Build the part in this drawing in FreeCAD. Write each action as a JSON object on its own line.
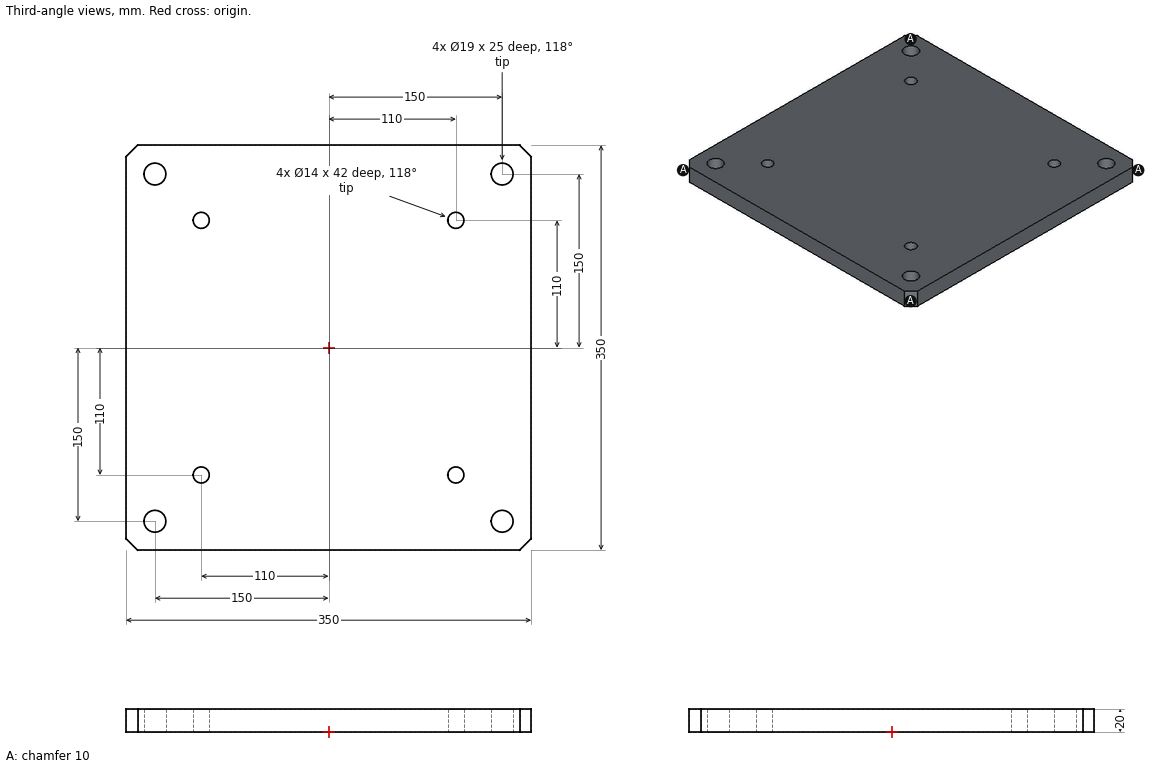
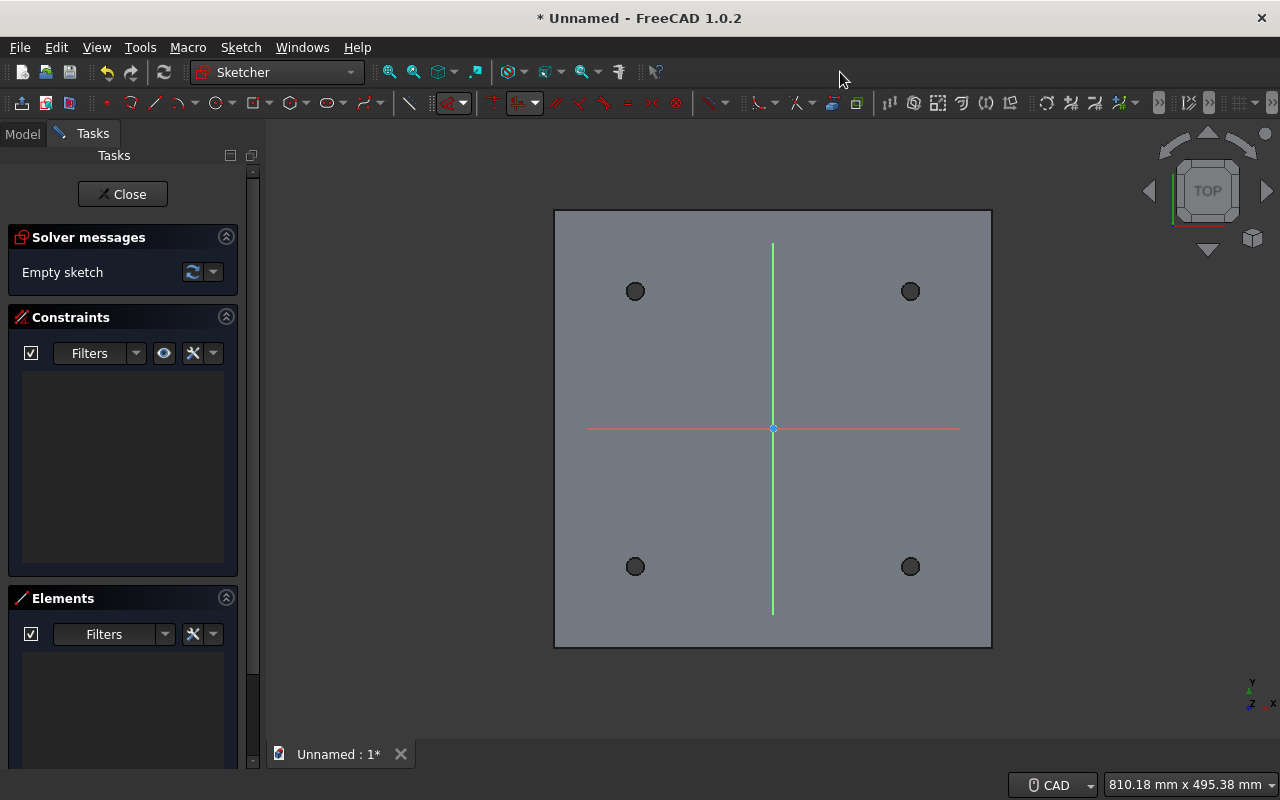
{"action": "left_click", "coordinate": [216, 104]}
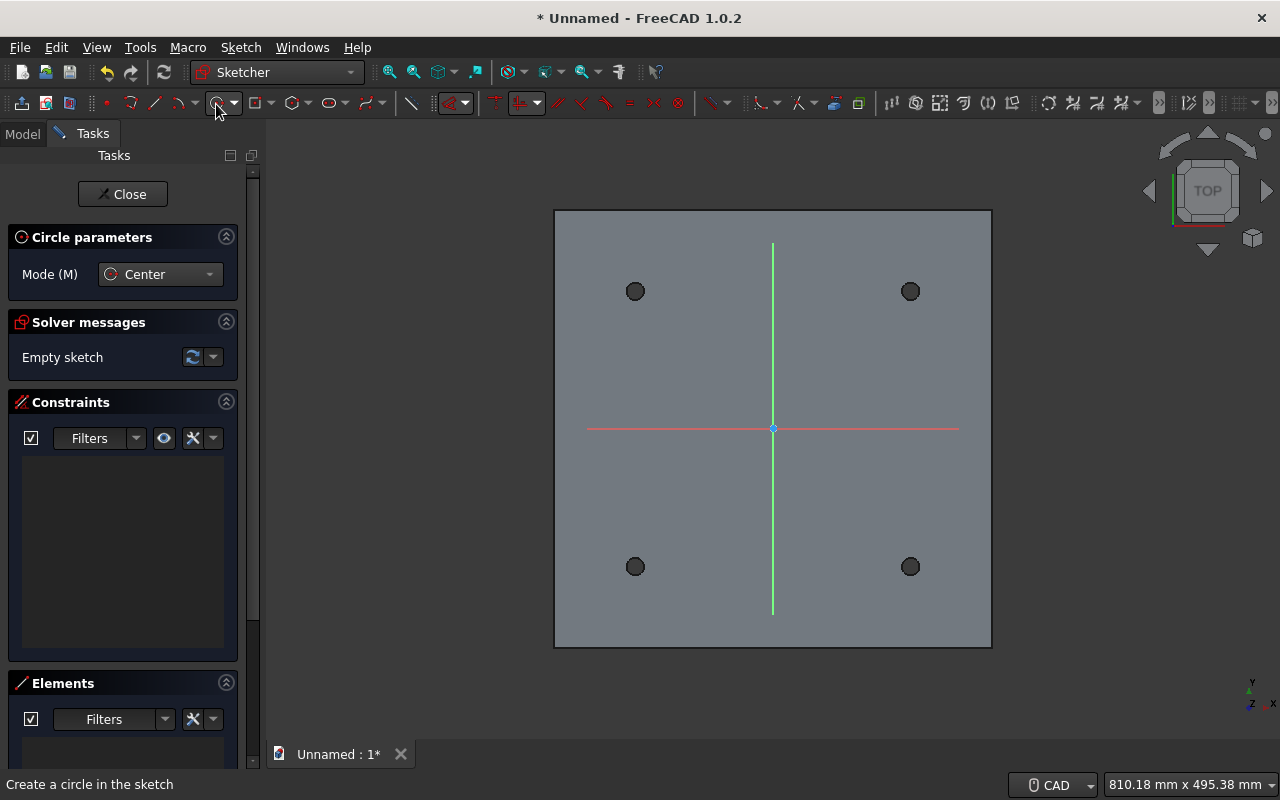
{"action": "scroll", "coordinate": [961, 241], "scroll_direction": "up", "scroll_amount": 4}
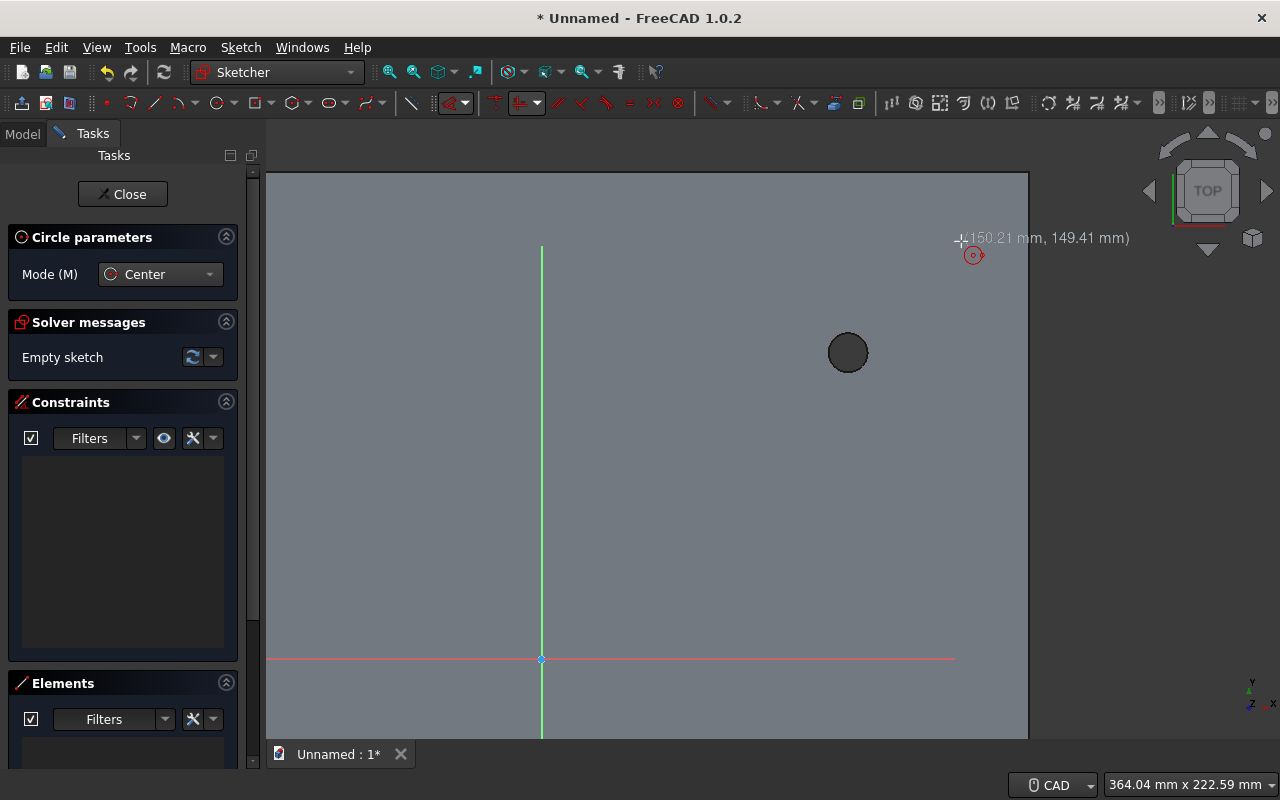
{"action": "left_click", "coordinate": [960, 241]}
{"action": "mouse_move", "coordinate": [978, 223]}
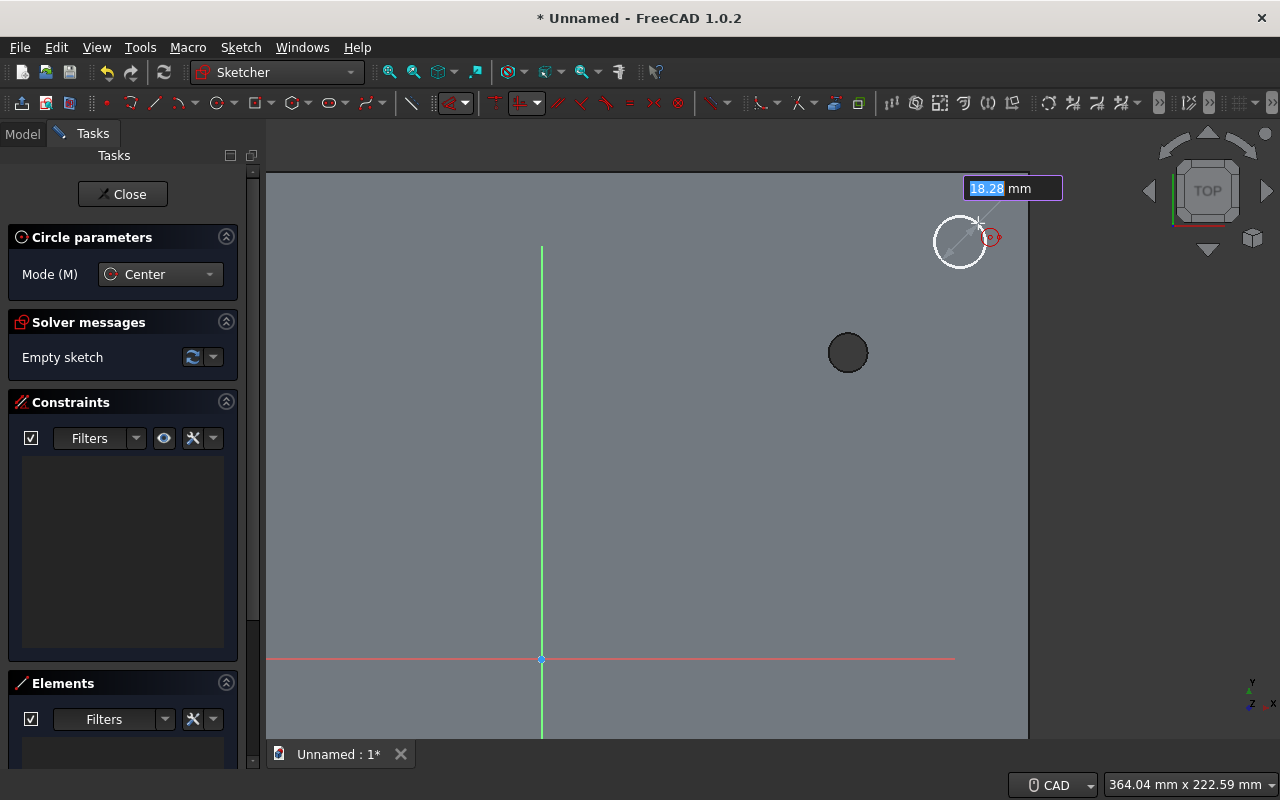
{"action": "type", "text": "19"}
{"action": "key", "text": "Return"}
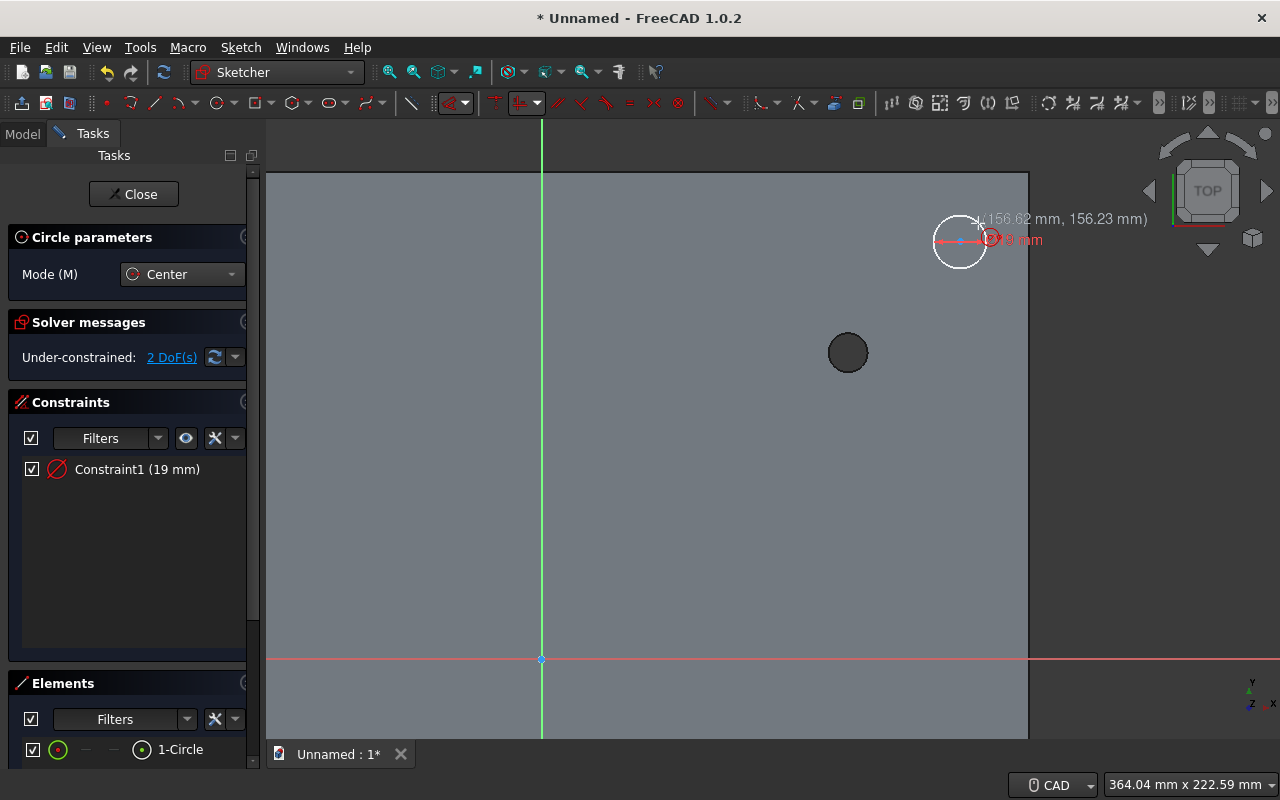
{"action": "scroll", "coordinate": [837, 241], "scroll_direction": "down", "scroll_amount": 4}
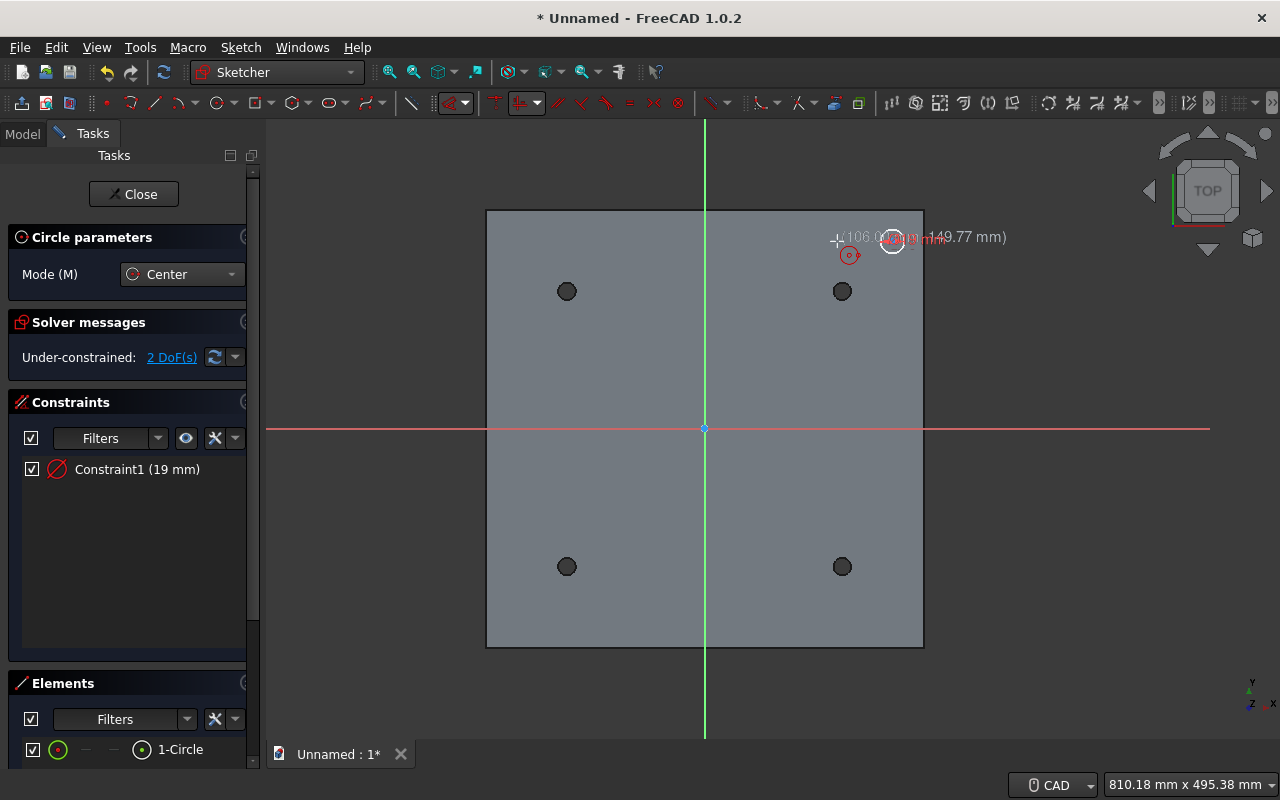
{"action": "scroll", "coordinate": [517, 617], "scroll_direction": "up", "scroll_amount": 4}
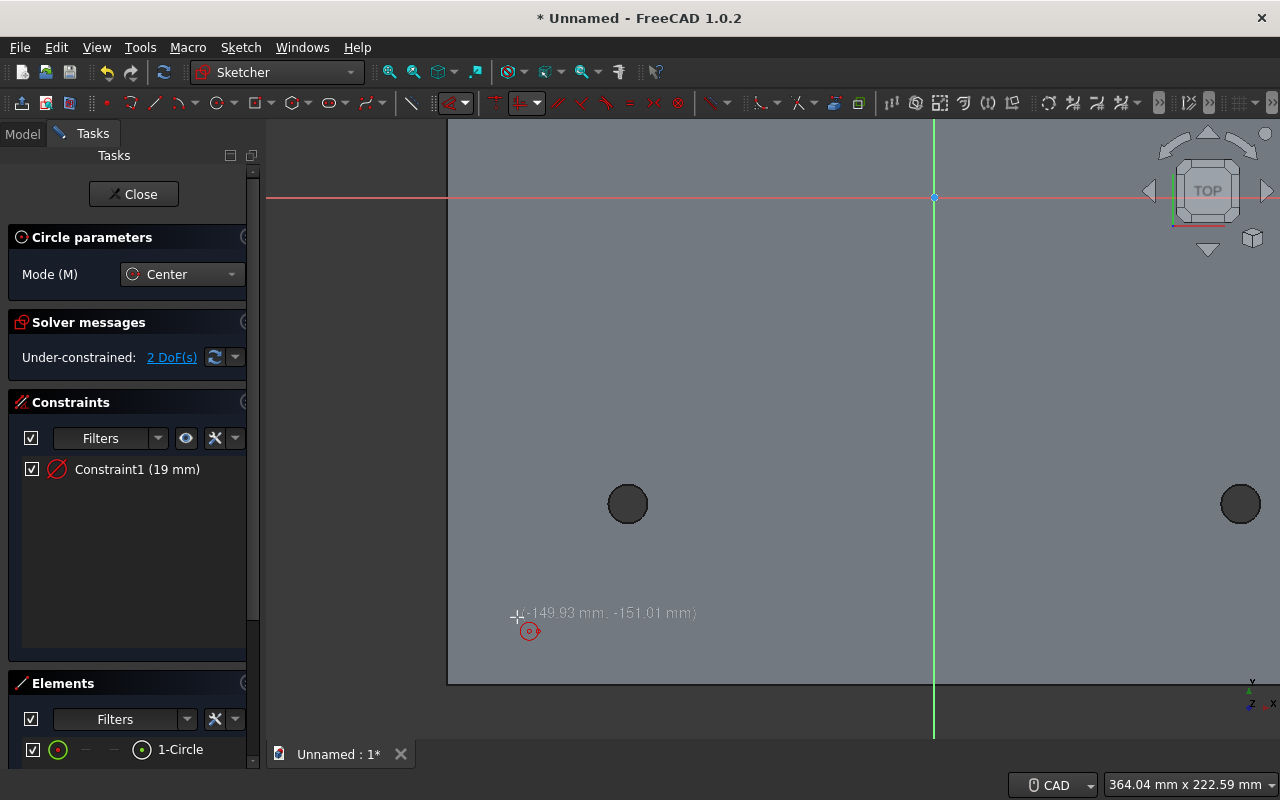
{"action": "left_click", "coordinate": [517, 615]}
{"action": "mouse_move", "coordinate": [535, 597]}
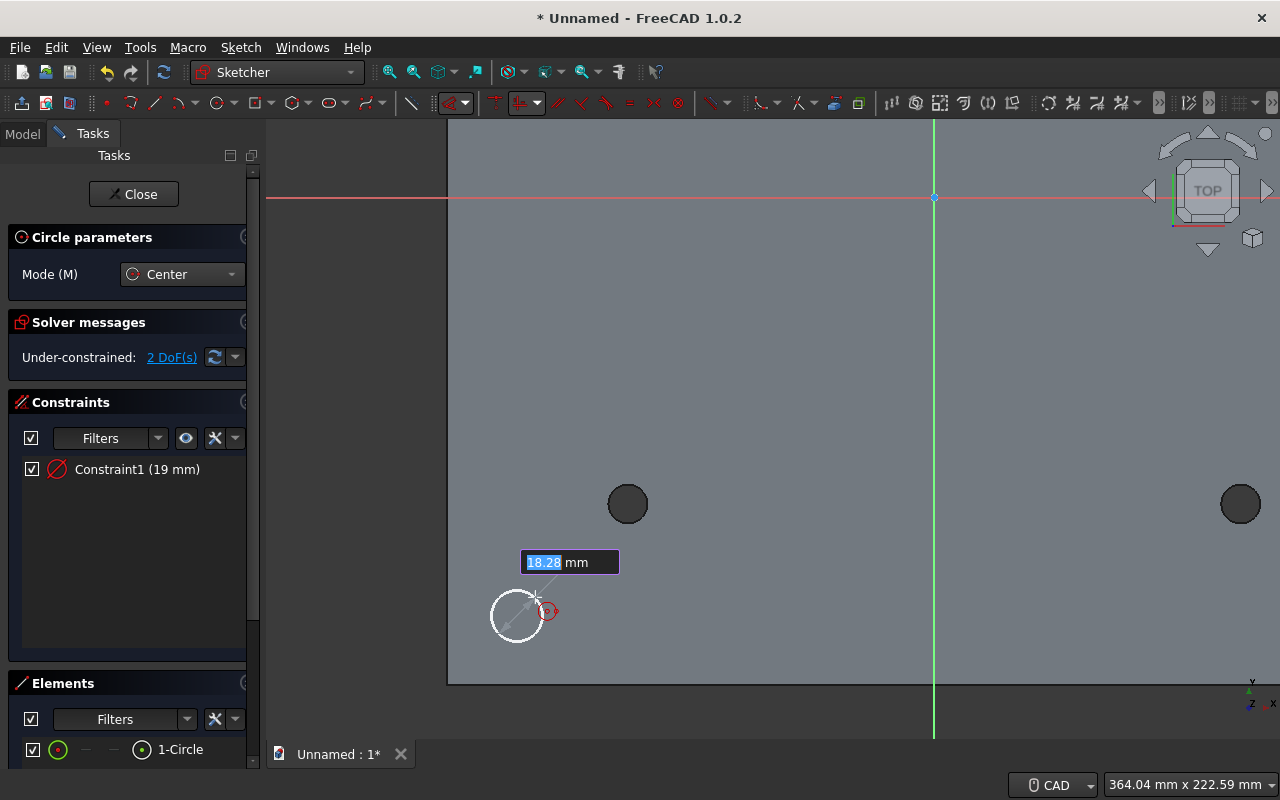
{"action": "type", "text": "19"}
{"action": "key", "text": "Return"}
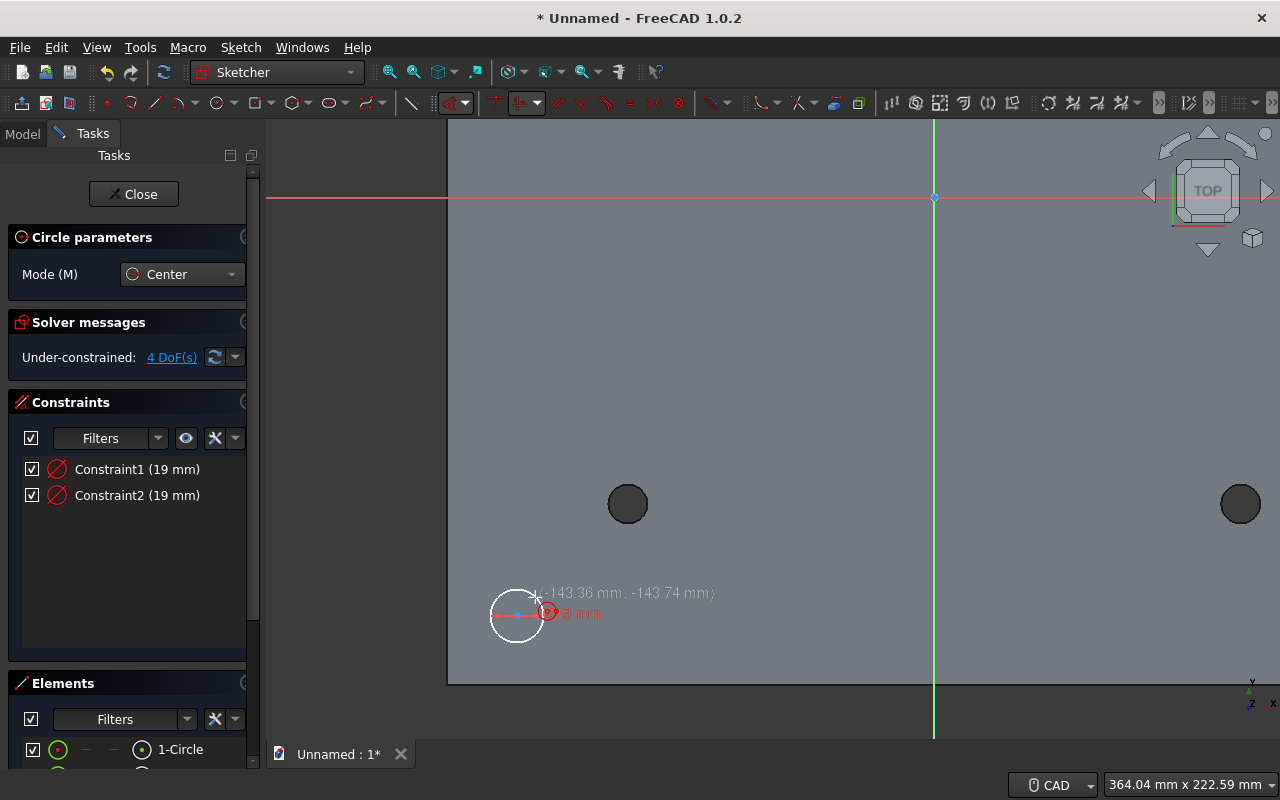
{"action": "scroll", "coordinate": [517, 618], "scroll_direction": "down", "scroll_amount": 4}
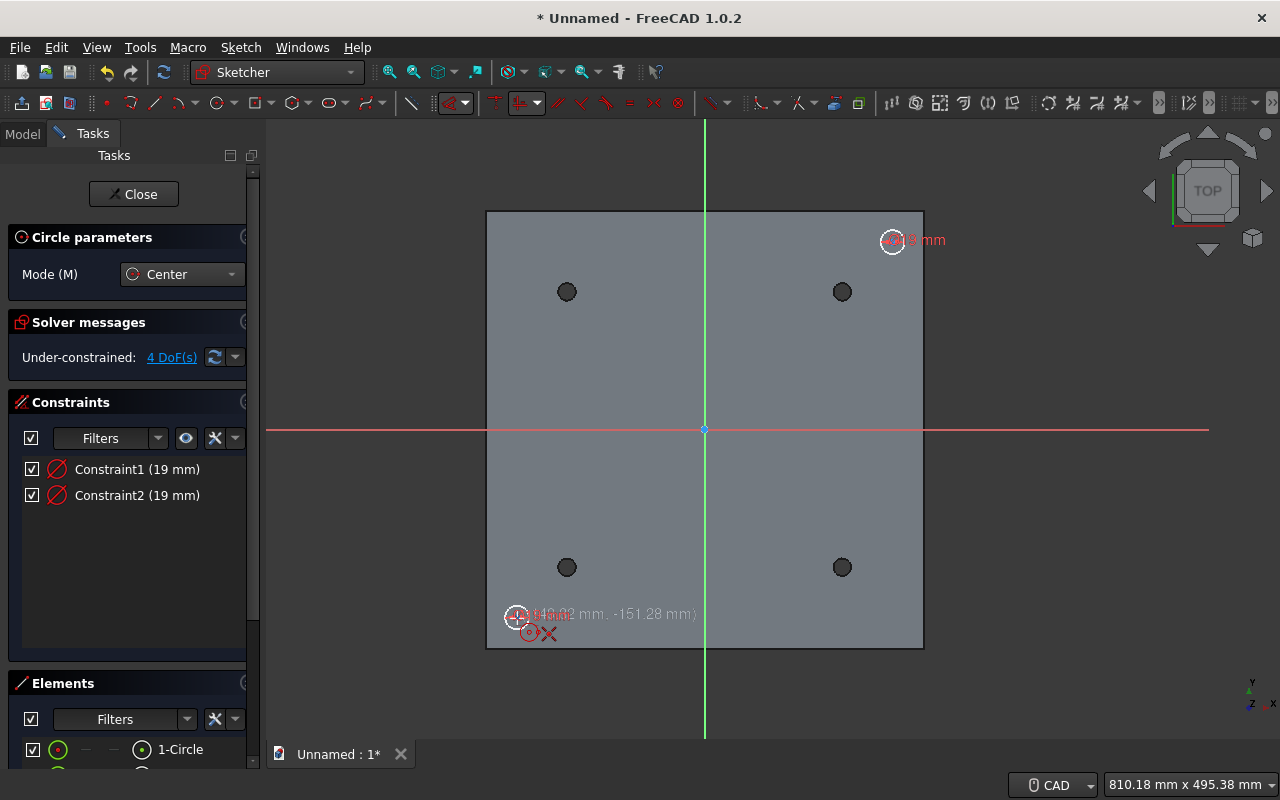
{"action": "scroll", "coordinate": [517, 242], "scroll_direction": "up", "scroll_amount": 4}